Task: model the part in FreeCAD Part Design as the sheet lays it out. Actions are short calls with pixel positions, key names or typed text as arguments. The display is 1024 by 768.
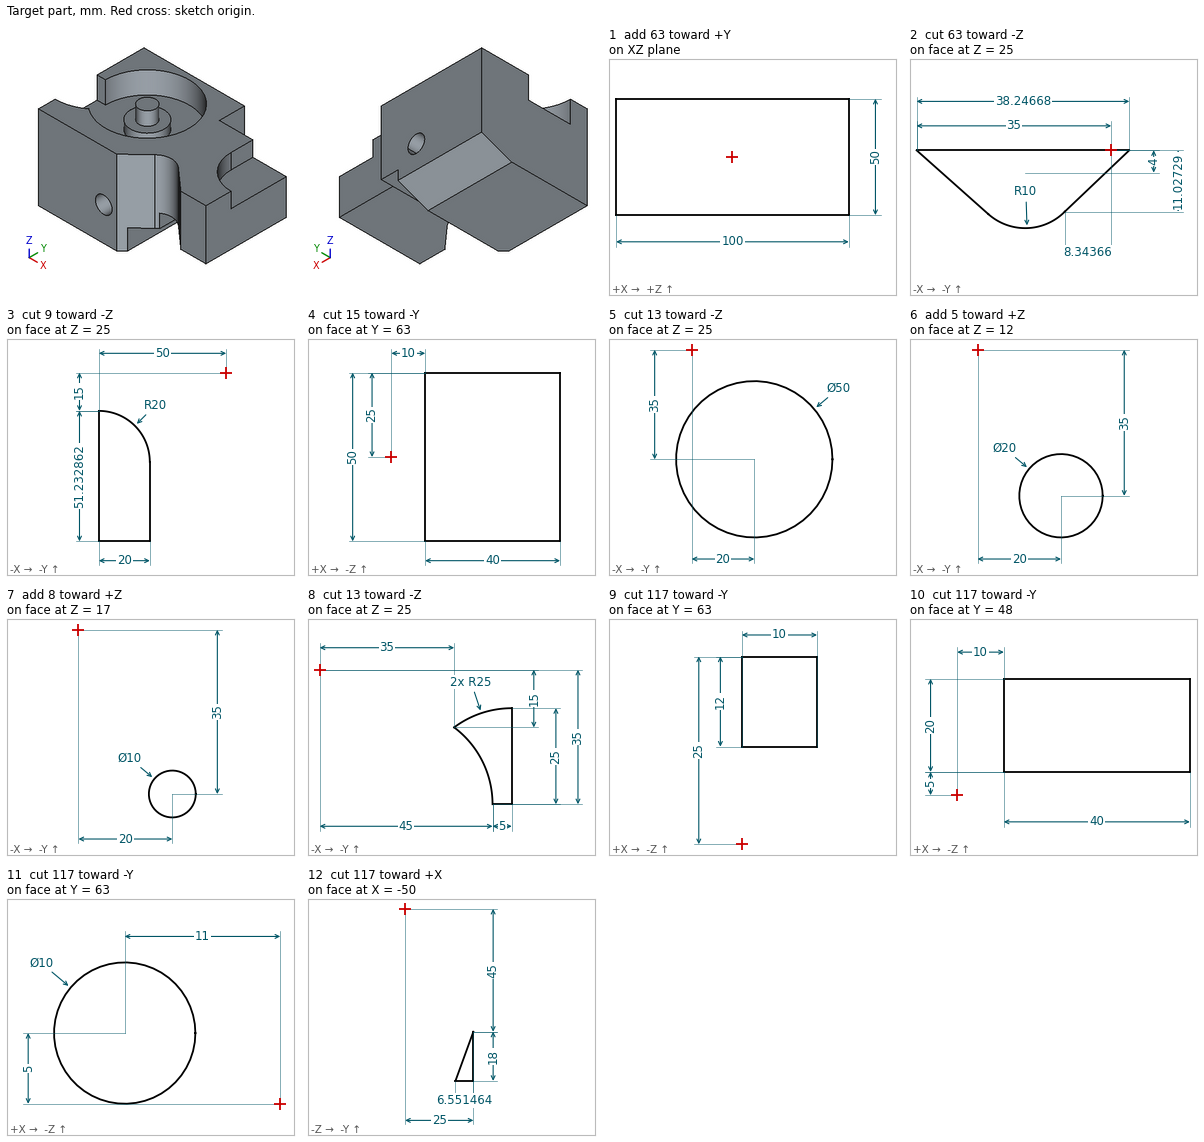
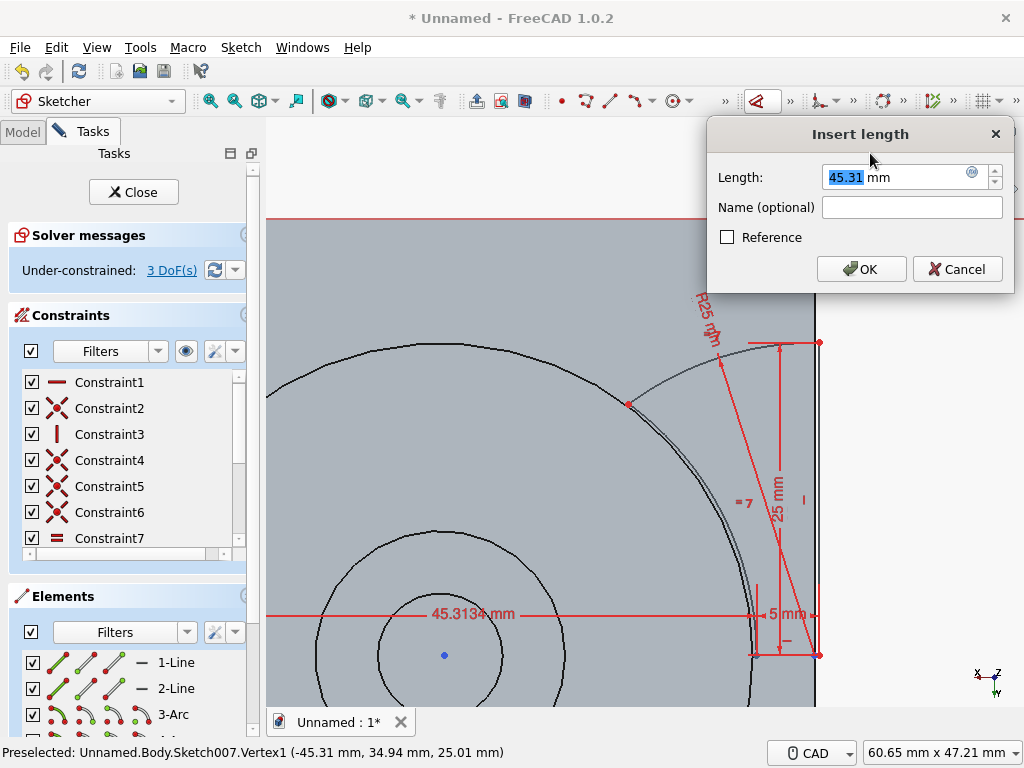
text(45)
key(Return)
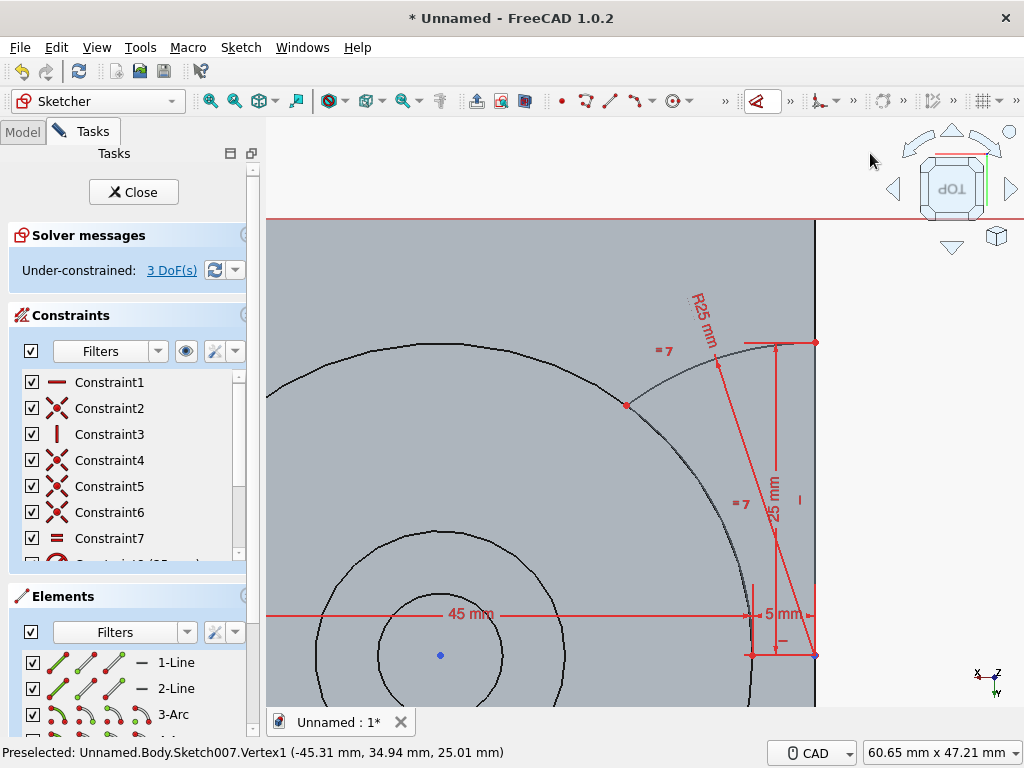
click(753, 655)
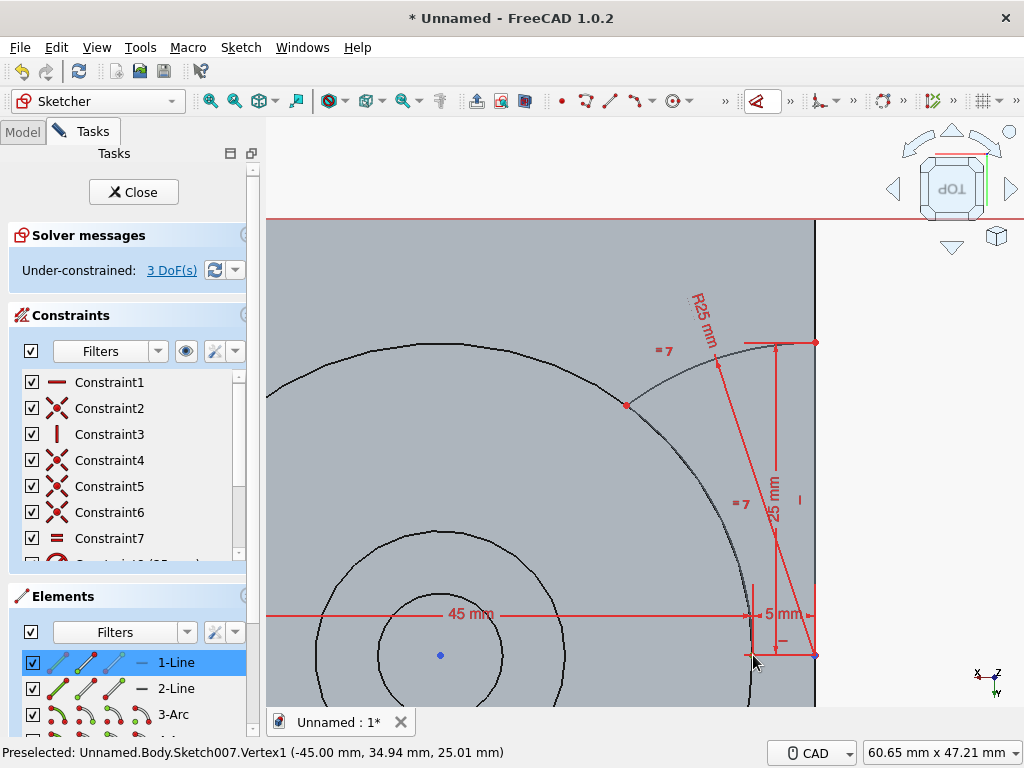
click(776, 102)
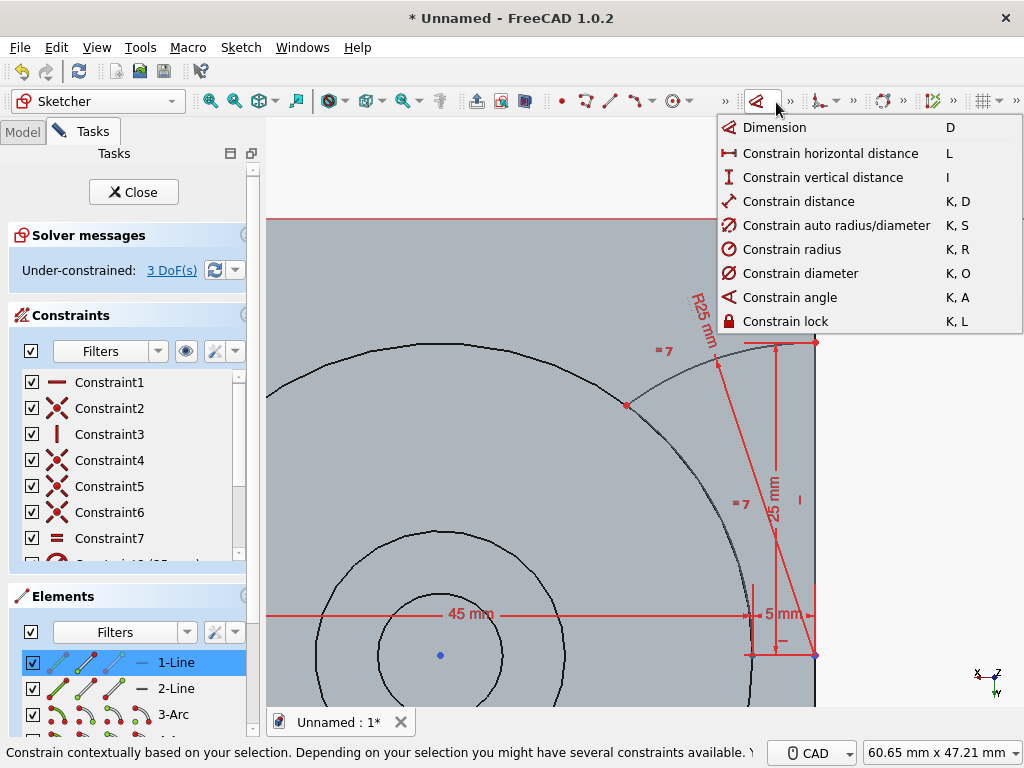
click(870, 177)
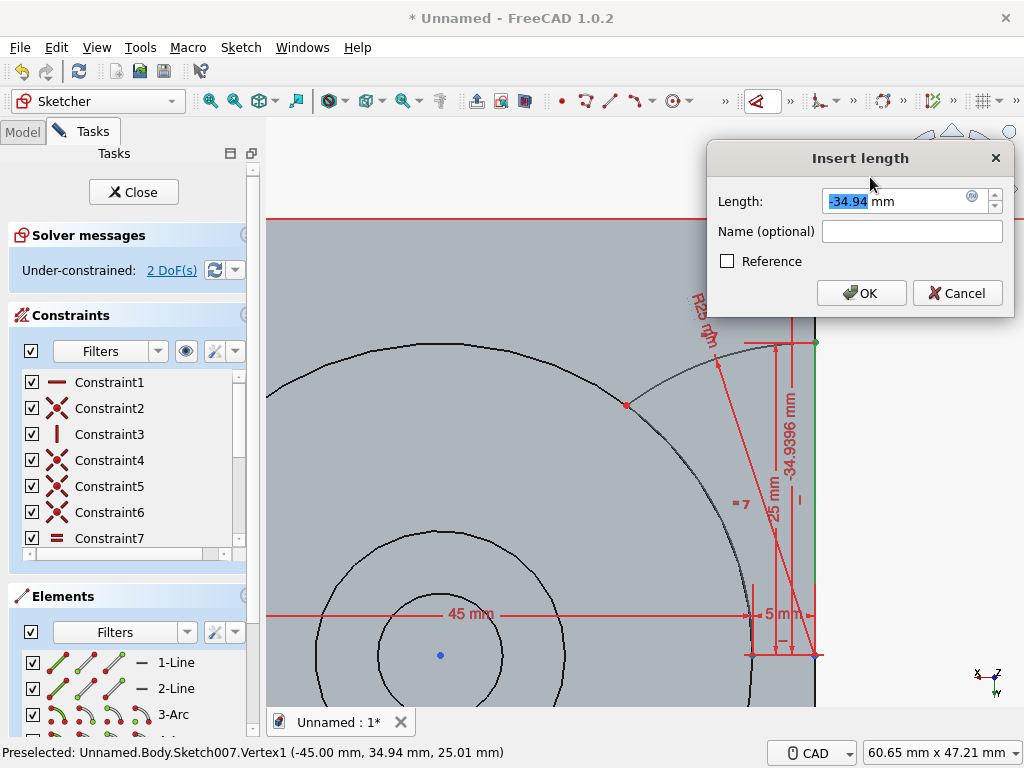
text(-35)
key(Return)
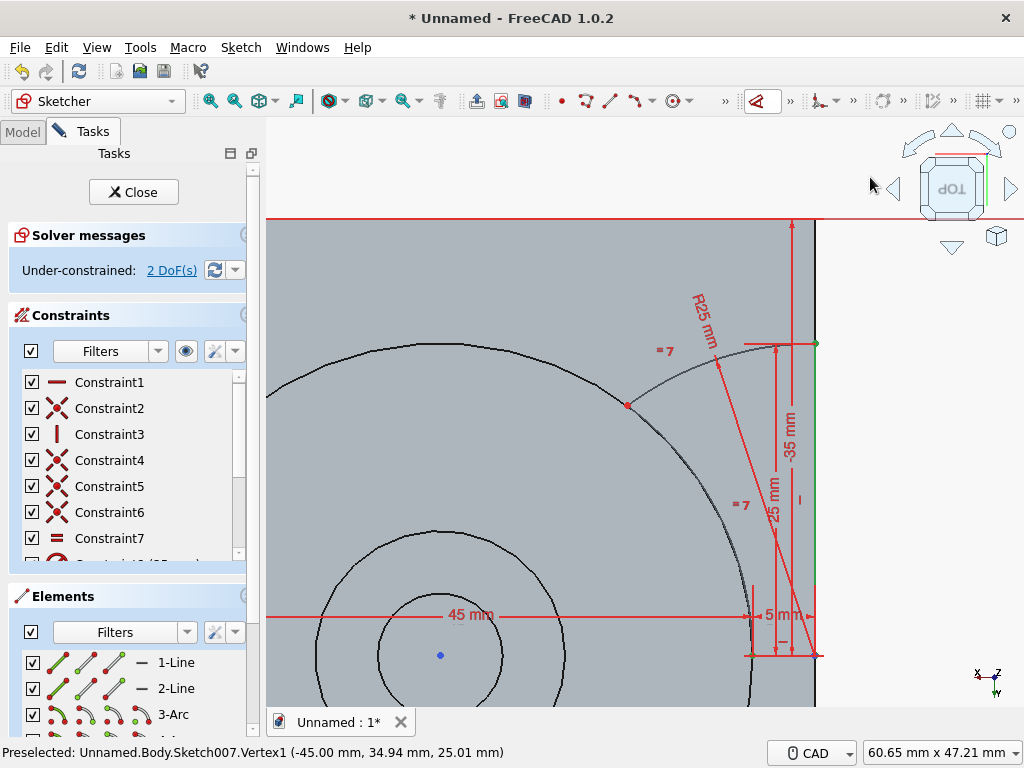
click(627, 406)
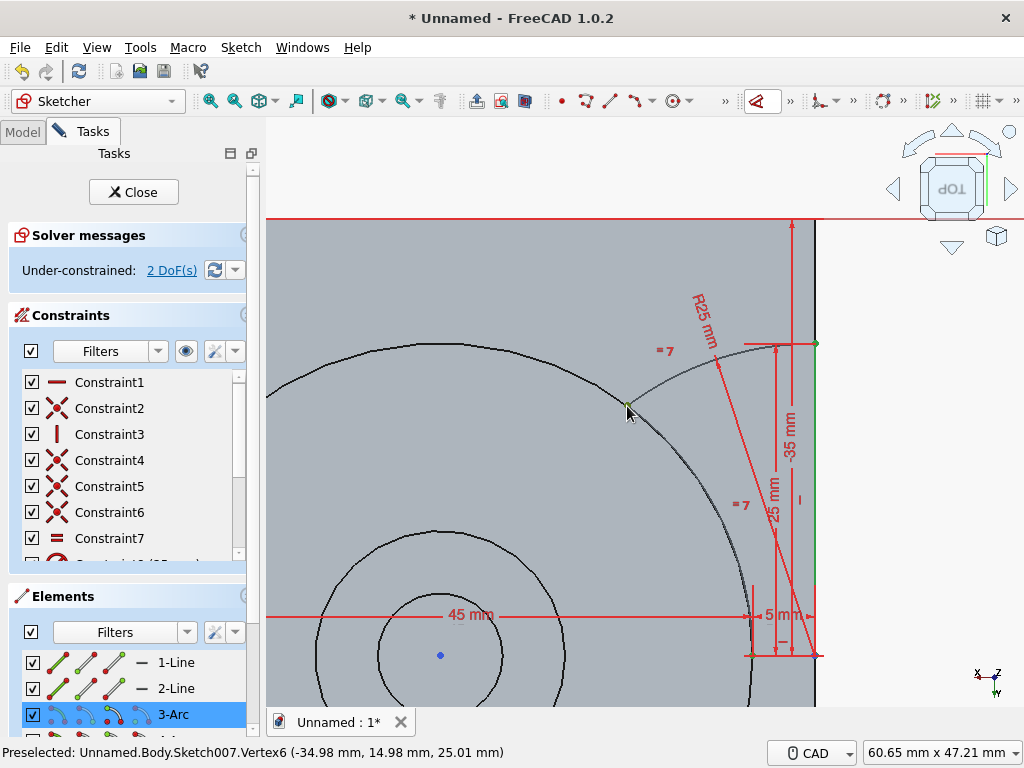
click(776, 102)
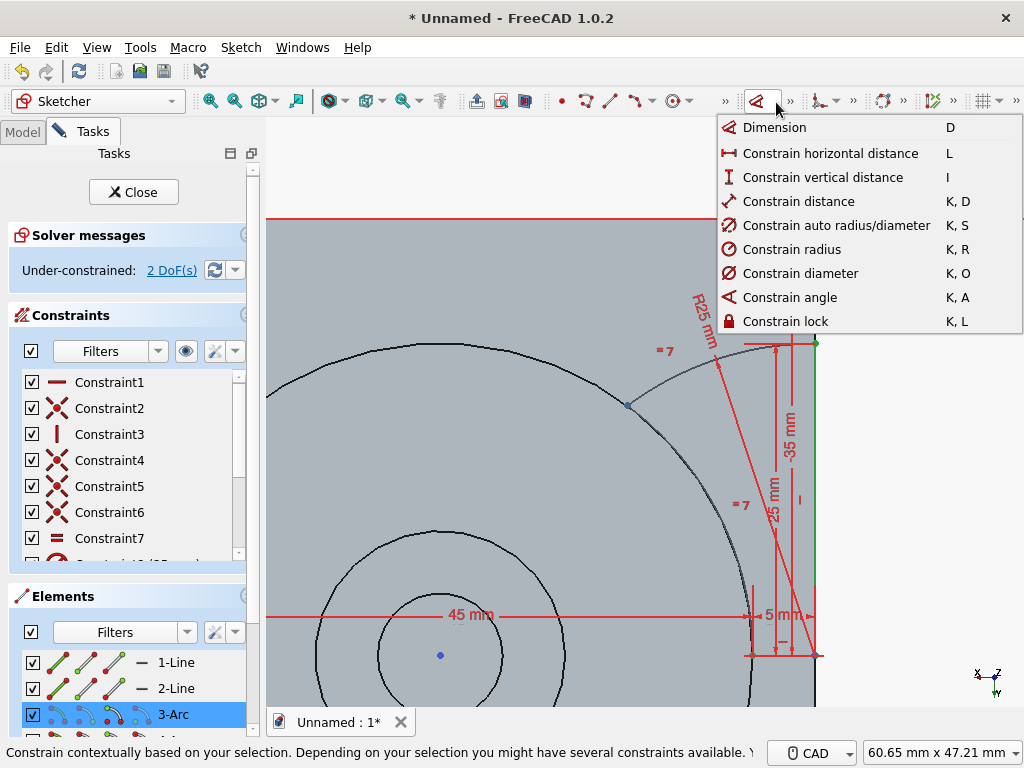
click(870, 153)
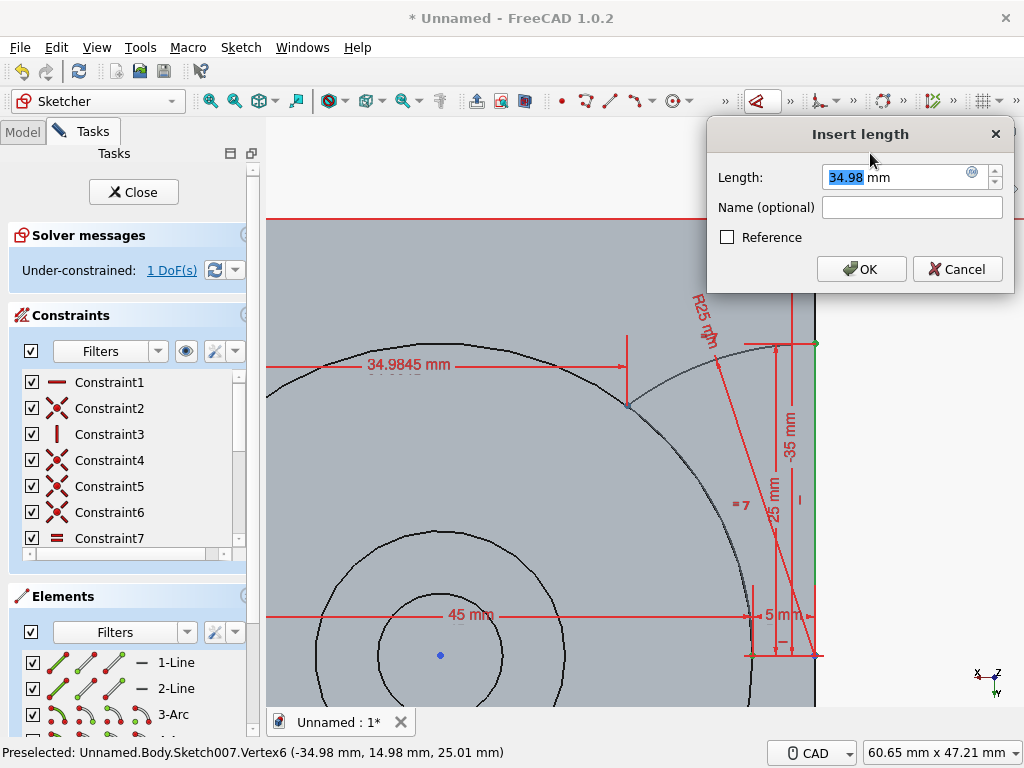
text(35)
key(Return)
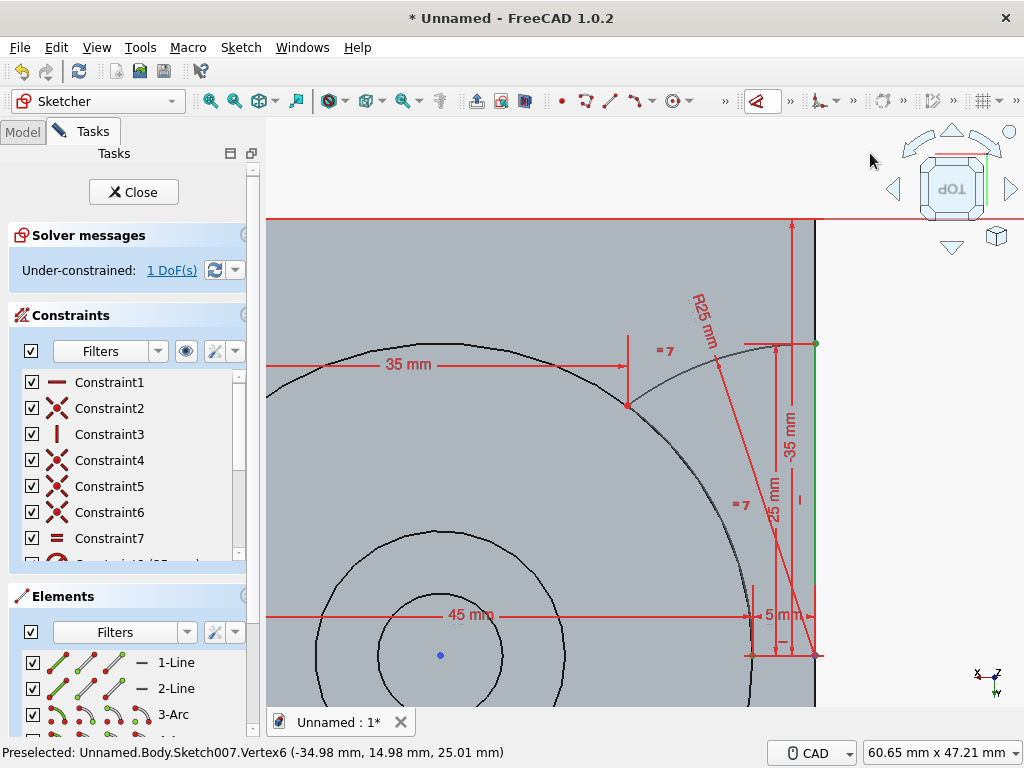
click(628, 406)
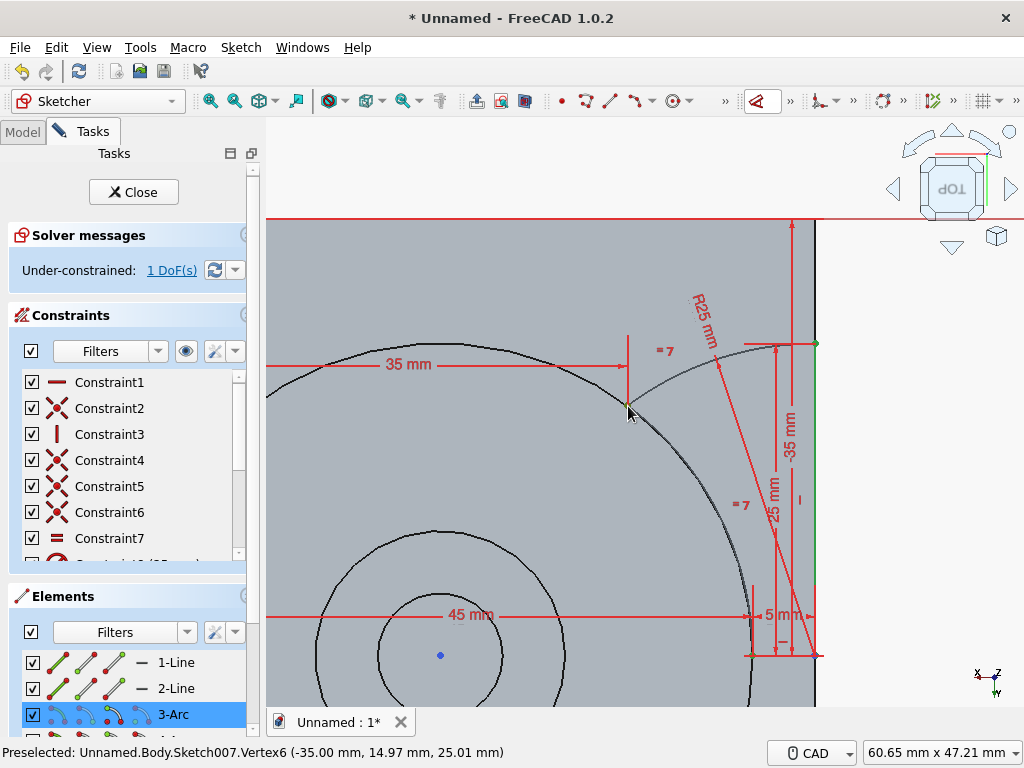
click(776, 102)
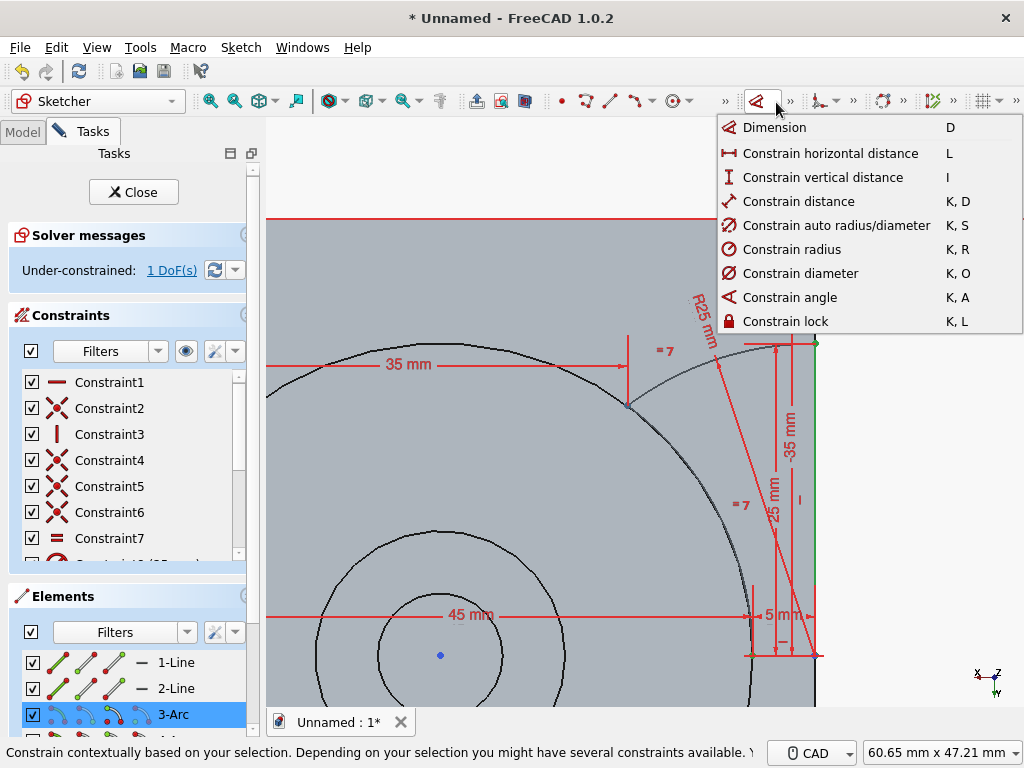
click(870, 177)